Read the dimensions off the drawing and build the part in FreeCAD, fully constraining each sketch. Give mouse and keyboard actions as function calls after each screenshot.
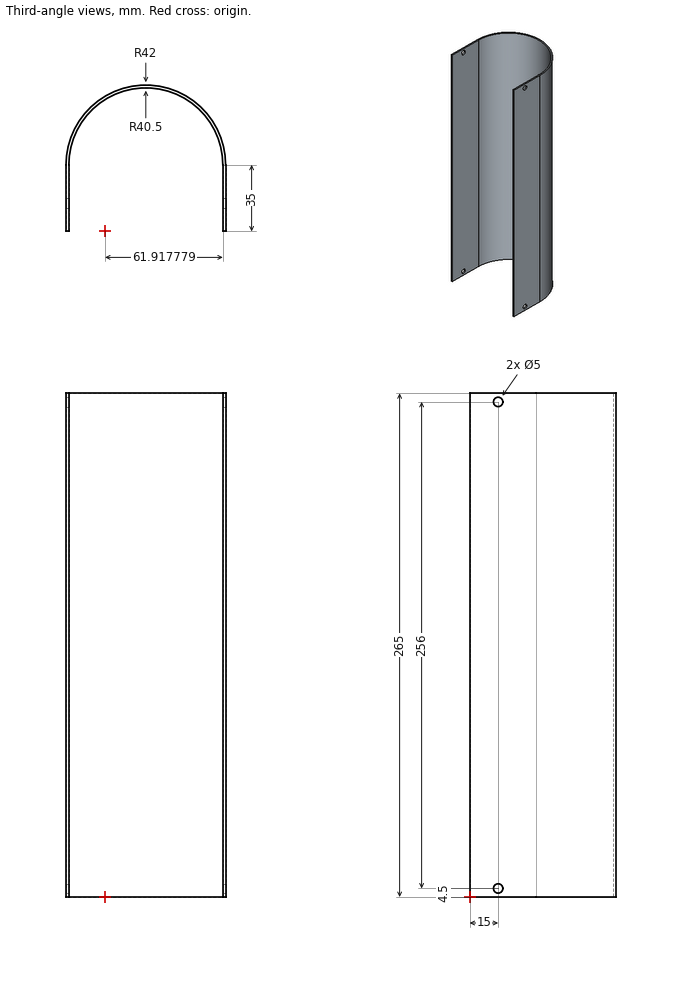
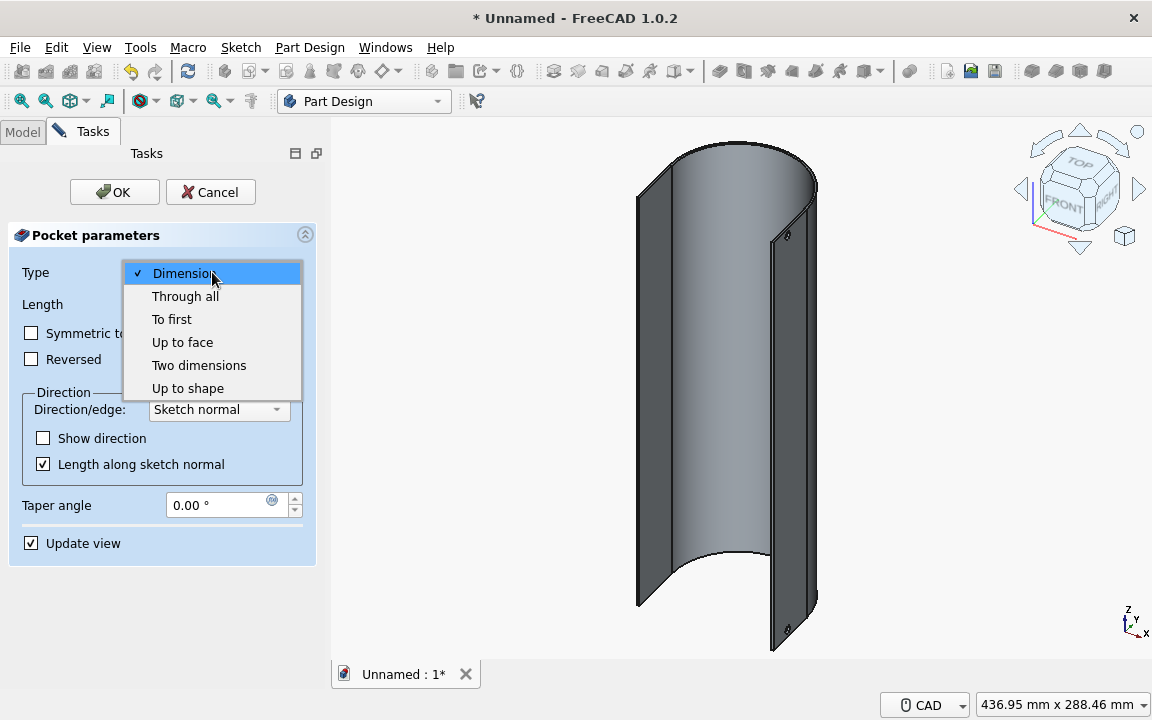
click(212, 296)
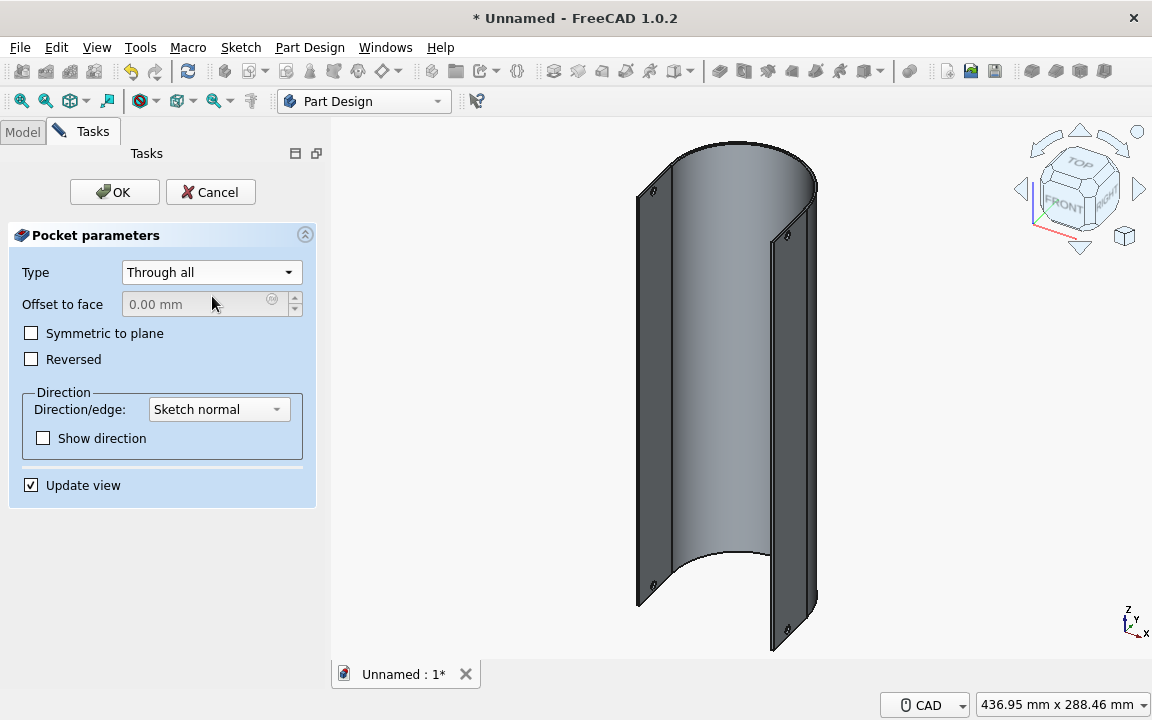
click(115, 192)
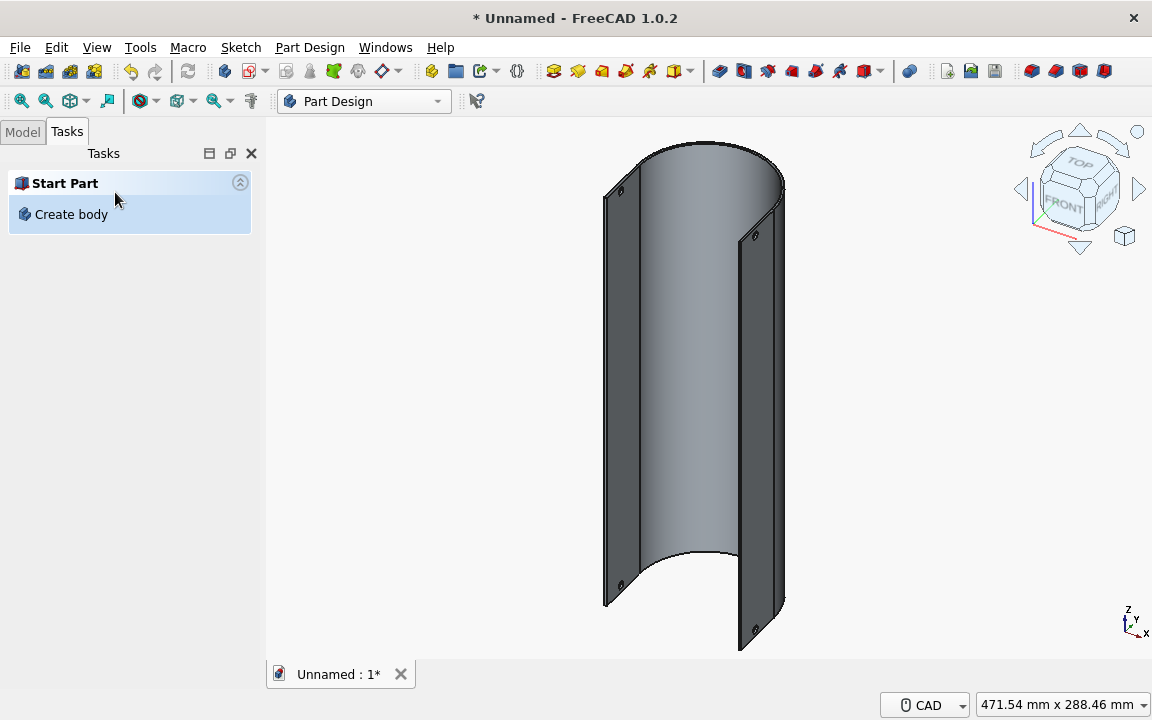
key(0)